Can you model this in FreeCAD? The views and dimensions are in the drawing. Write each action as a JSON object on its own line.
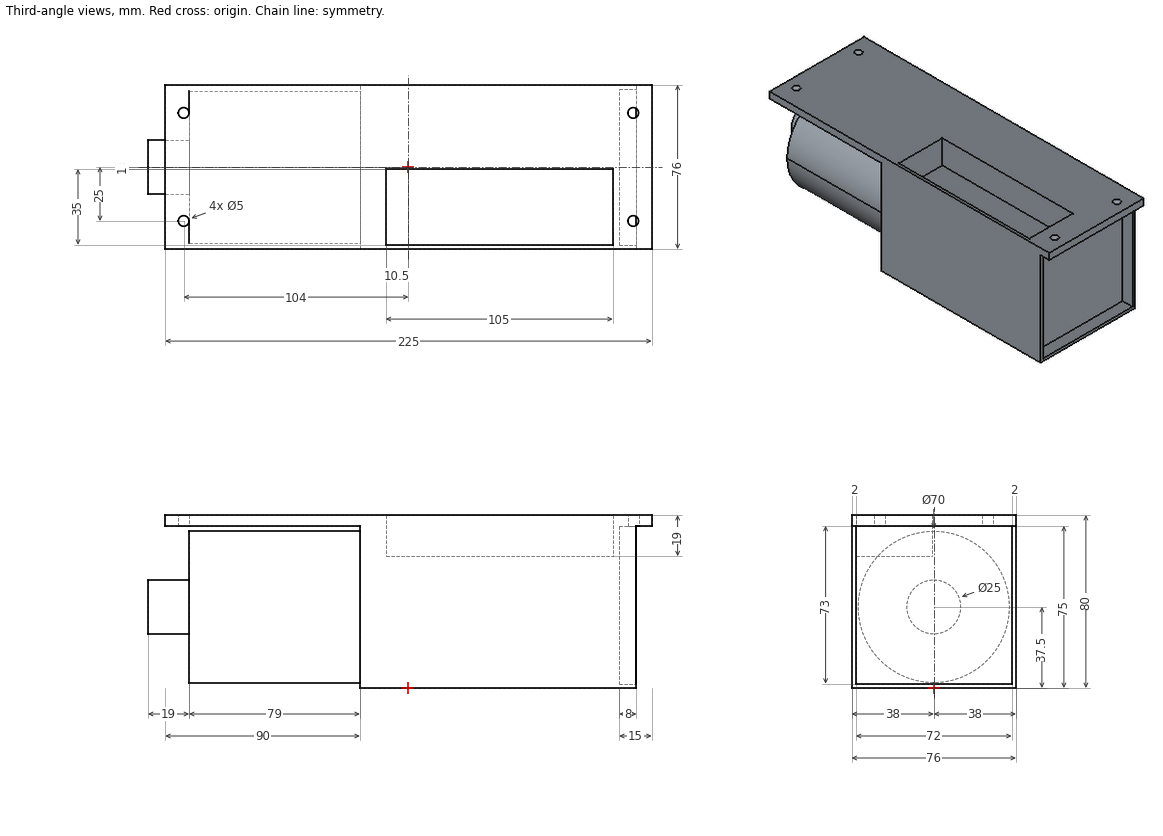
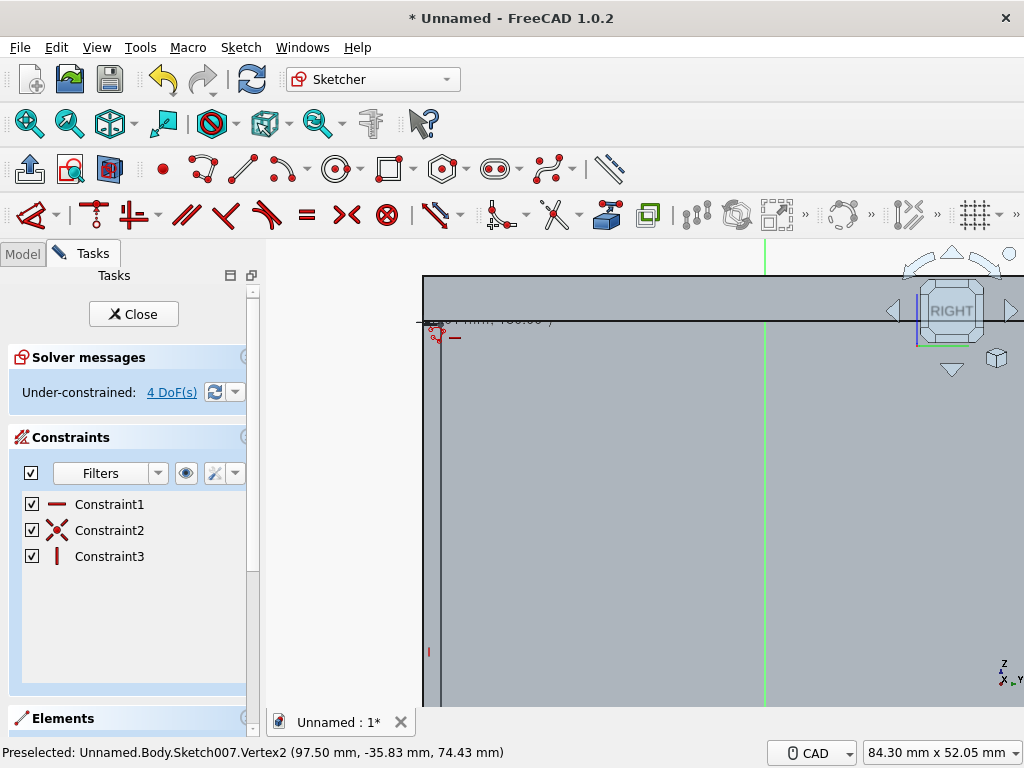
{"action": "left_click", "coordinate": [423, 322]}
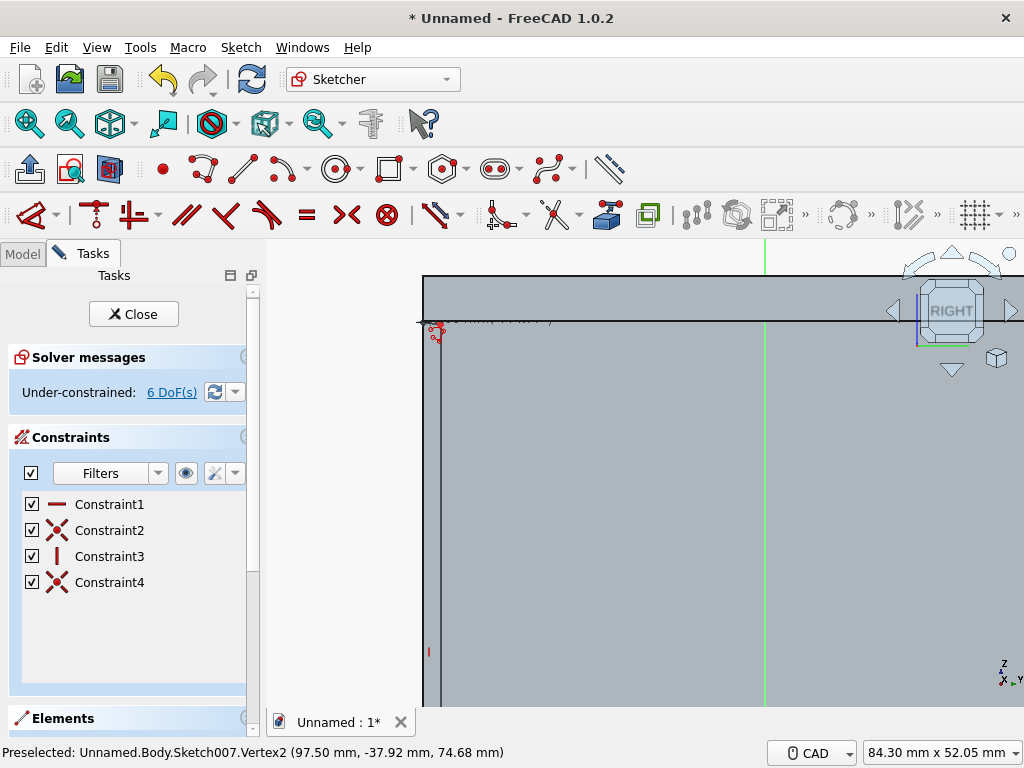
{"action": "scroll", "coordinate": [423, 322], "scroll_direction": "down", "scroll_amount": 4}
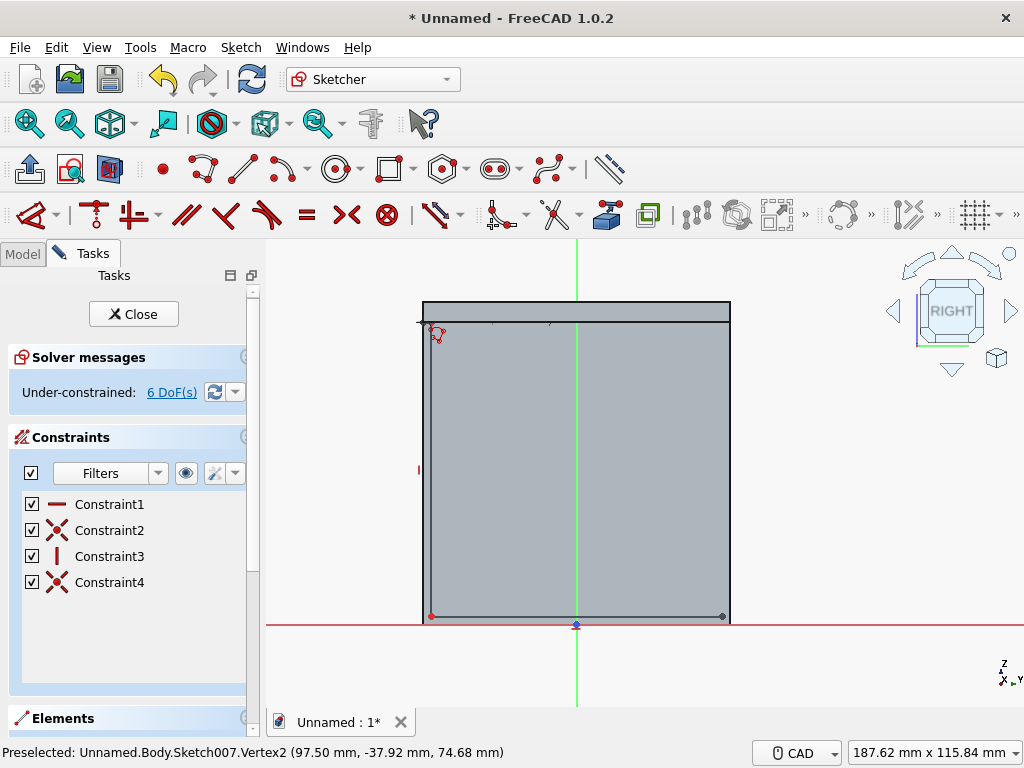
{"action": "scroll", "coordinate": [423, 625], "scroll_direction": "up", "scroll_amount": 2}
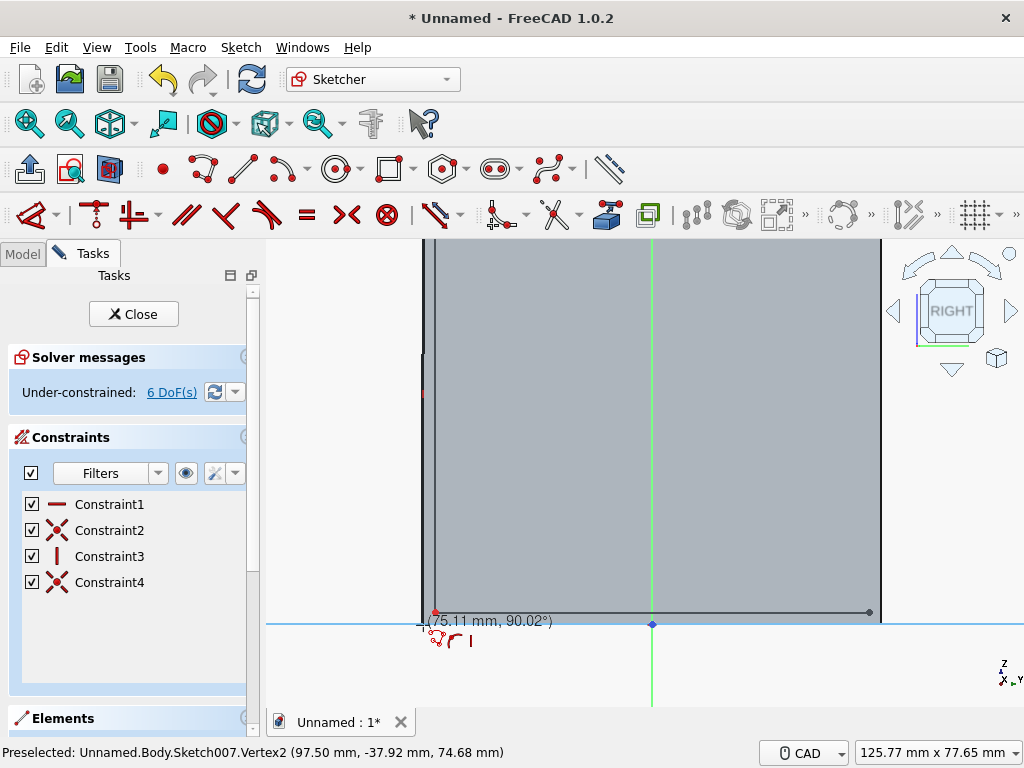
{"action": "left_click", "coordinate": [423, 624]}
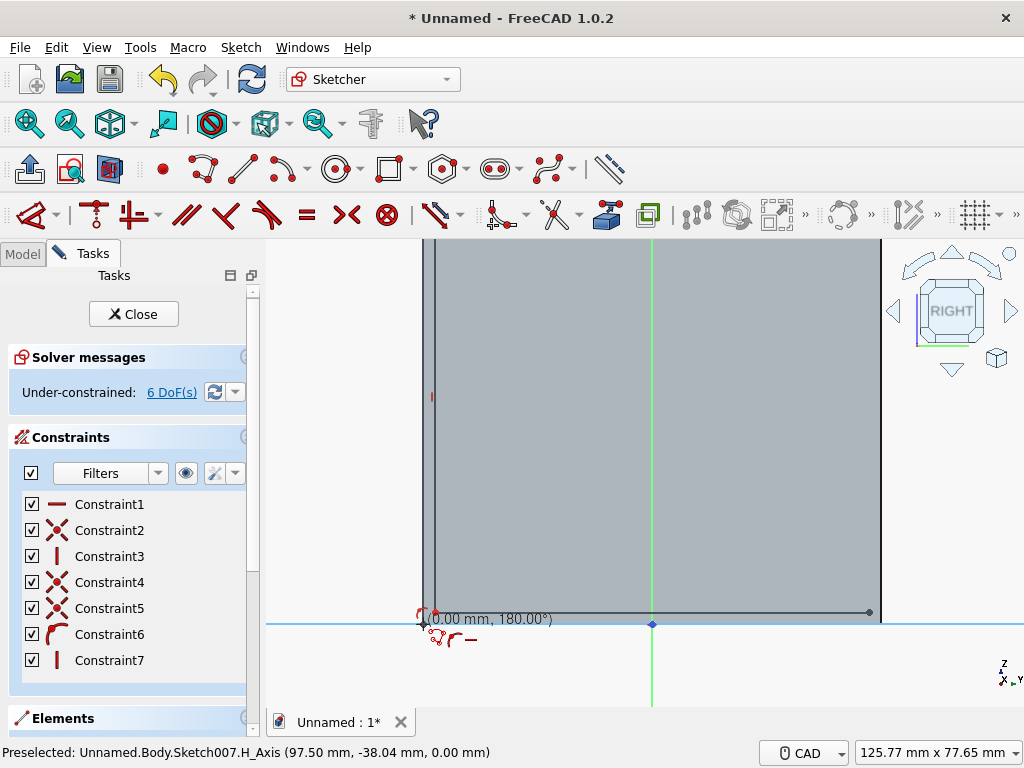
{"action": "scroll", "coordinate": [422, 625], "scroll_direction": "down", "scroll_amount": 2}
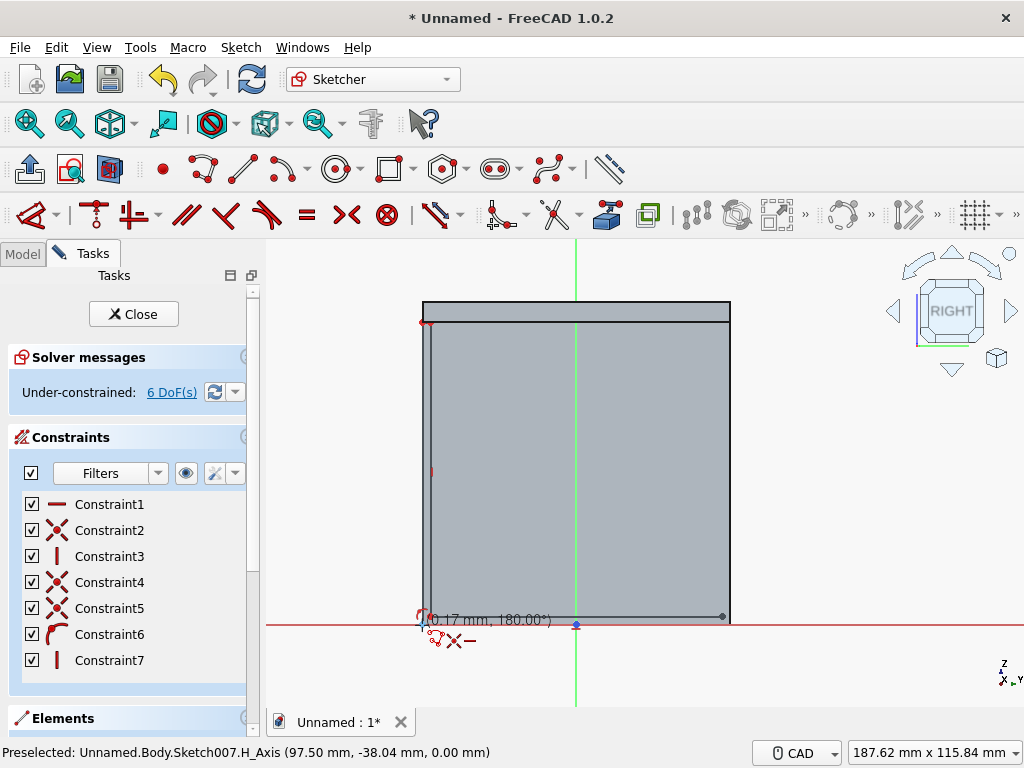
{"action": "scroll", "coordinate": [730, 625], "scroll_direction": "up", "scroll_amount": 2}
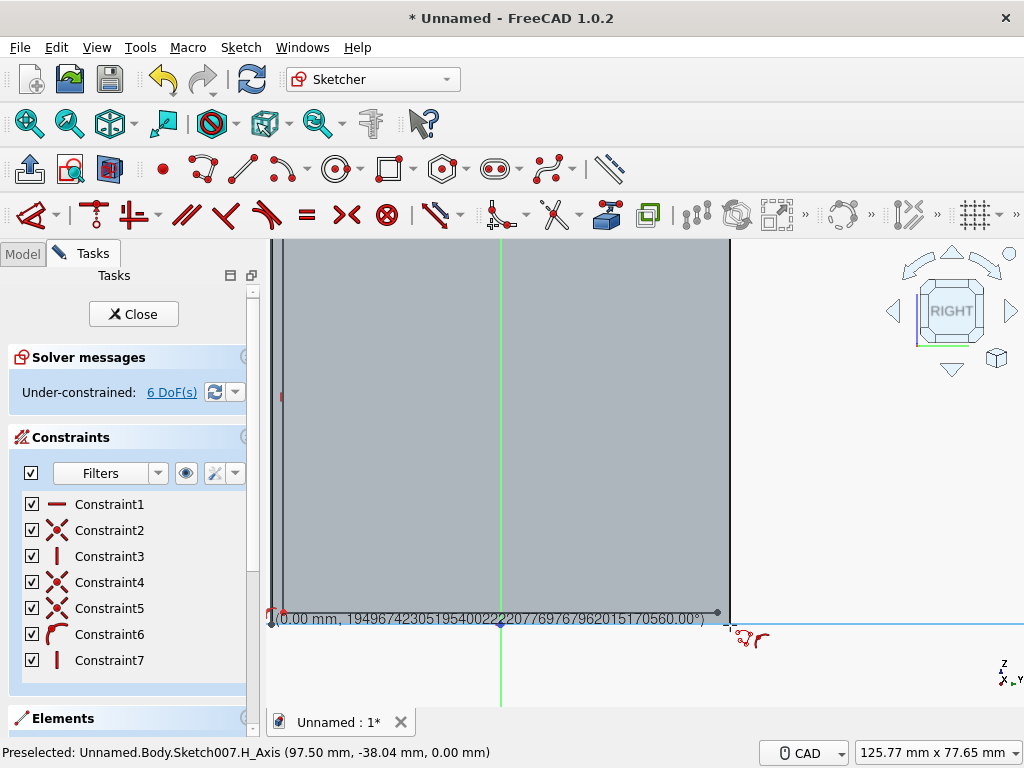
{"action": "left_click", "coordinate": [730, 615]}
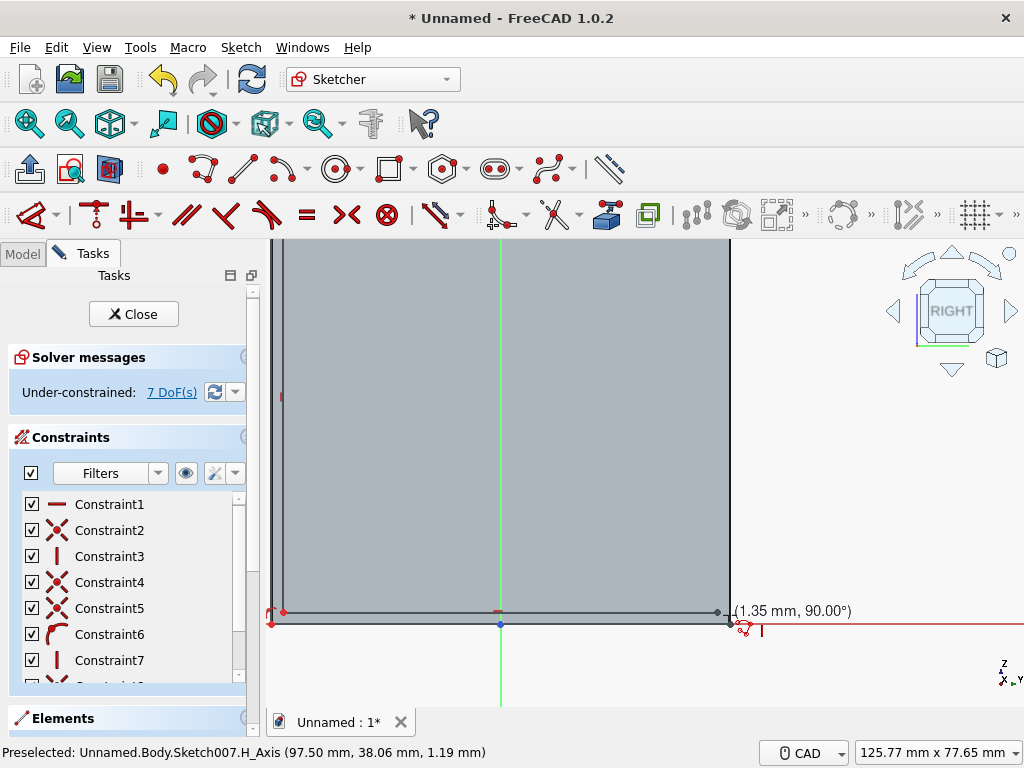
{"action": "scroll", "coordinate": [731, 625], "scroll_direction": "down", "scroll_amount": 2}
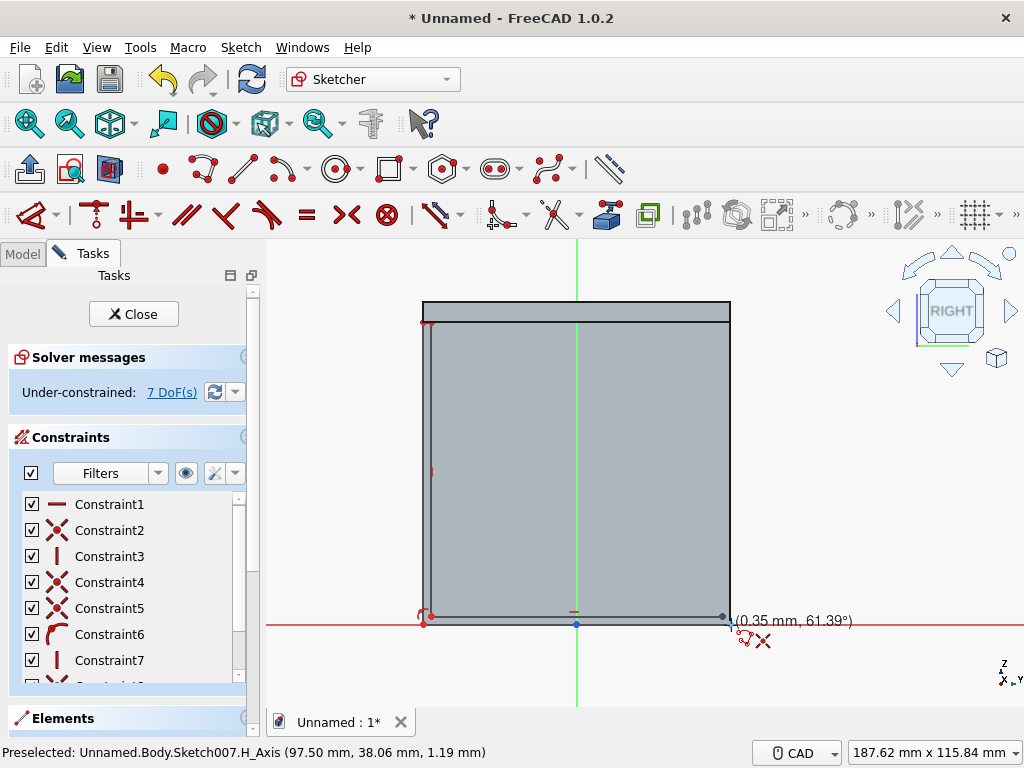
{"action": "left_click", "coordinate": [731, 322]}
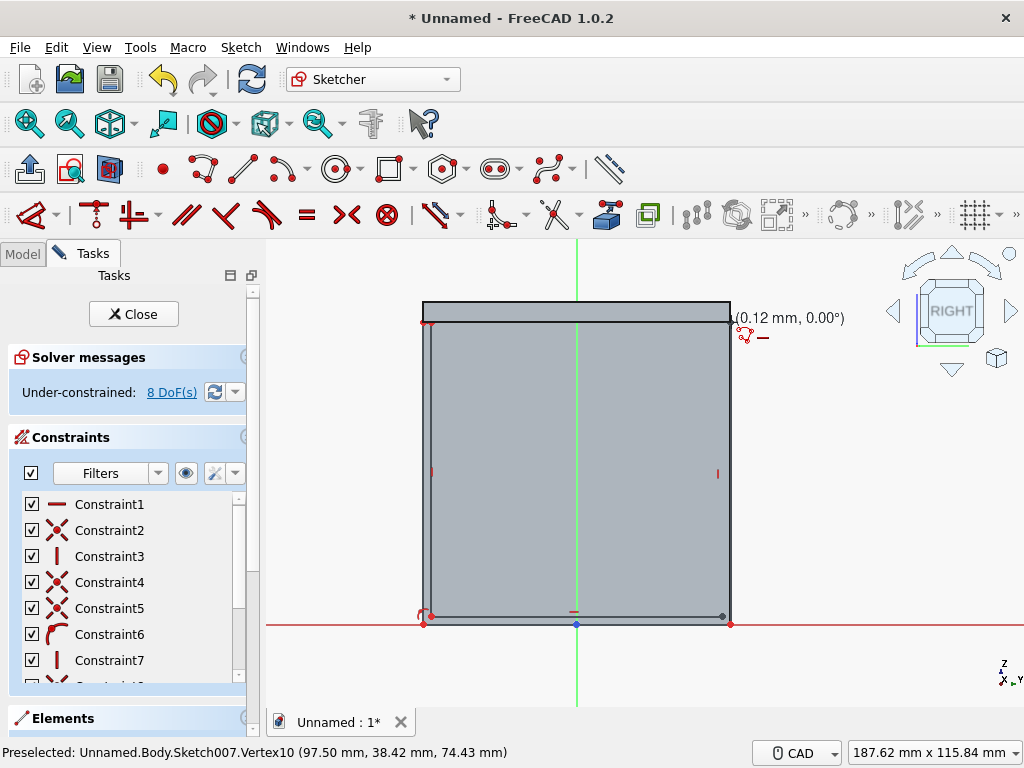
{"action": "scroll", "coordinate": [722, 322], "scroll_direction": "up", "scroll_amount": 4}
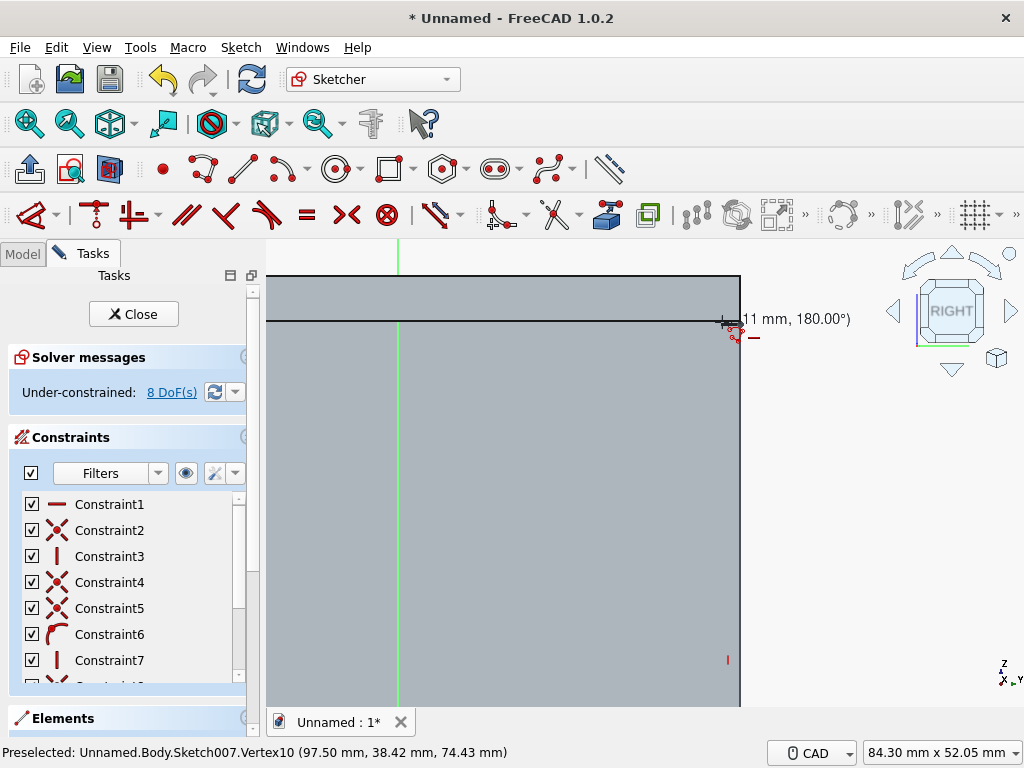
{"action": "left_click", "coordinate": [722, 322]}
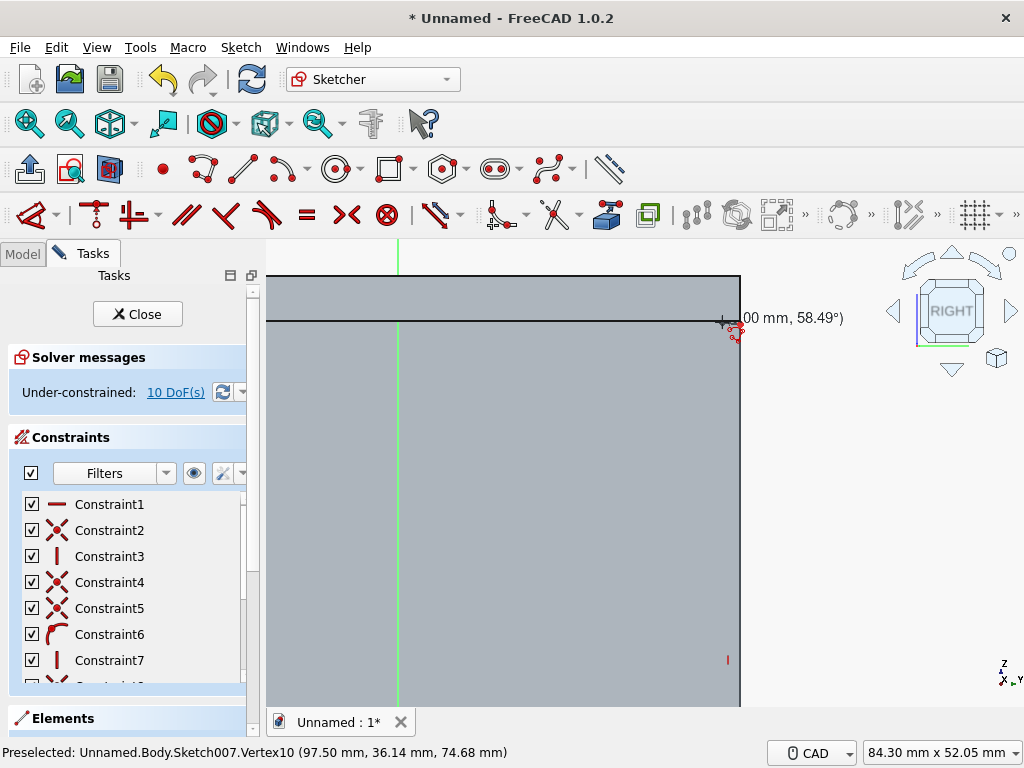
{"action": "scroll", "coordinate": [722, 322], "scroll_direction": "down", "scroll_amount": 4}